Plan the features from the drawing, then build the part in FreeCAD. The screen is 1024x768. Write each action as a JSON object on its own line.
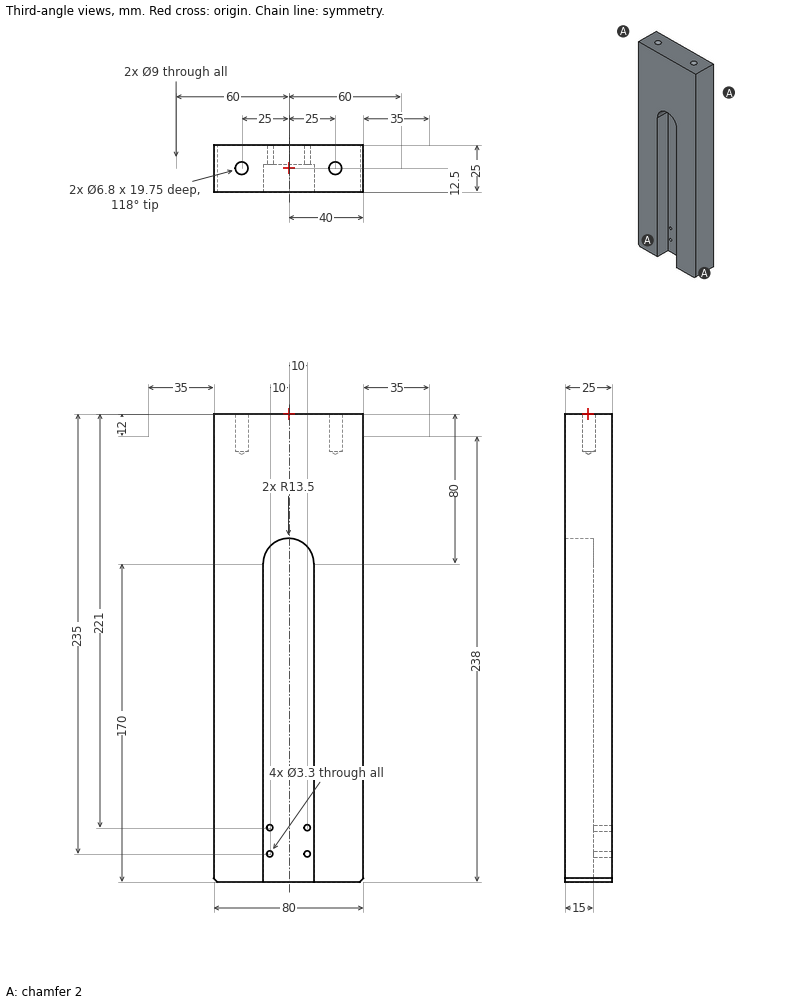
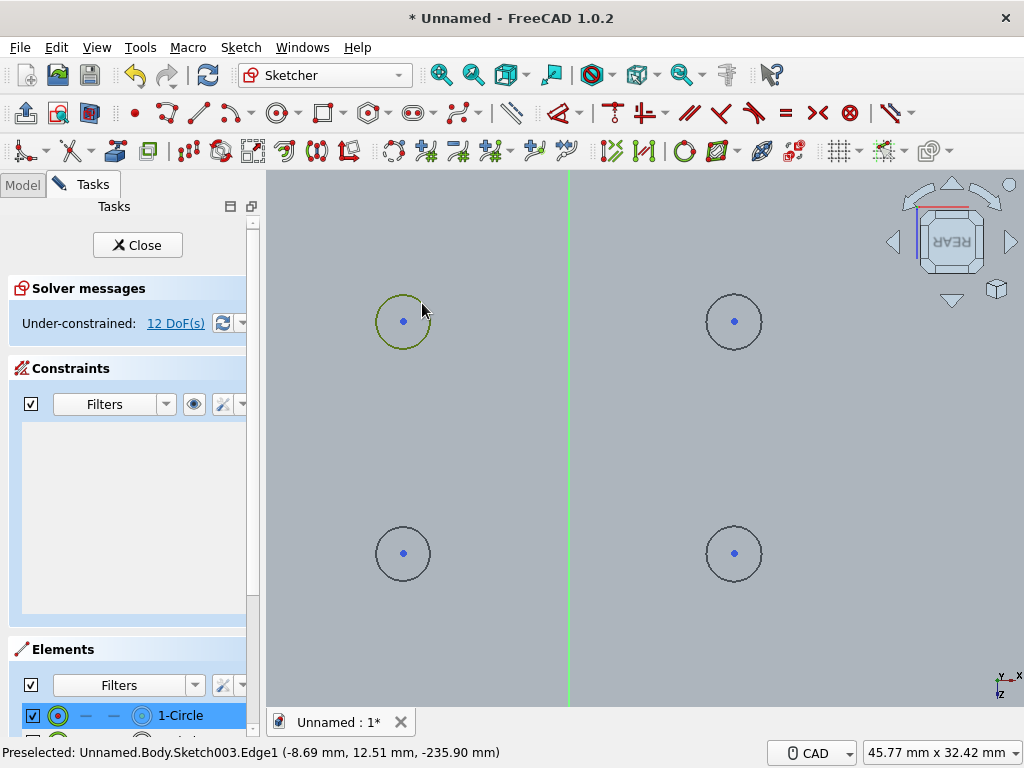
{"action": "left_click", "coordinate": [422, 535]}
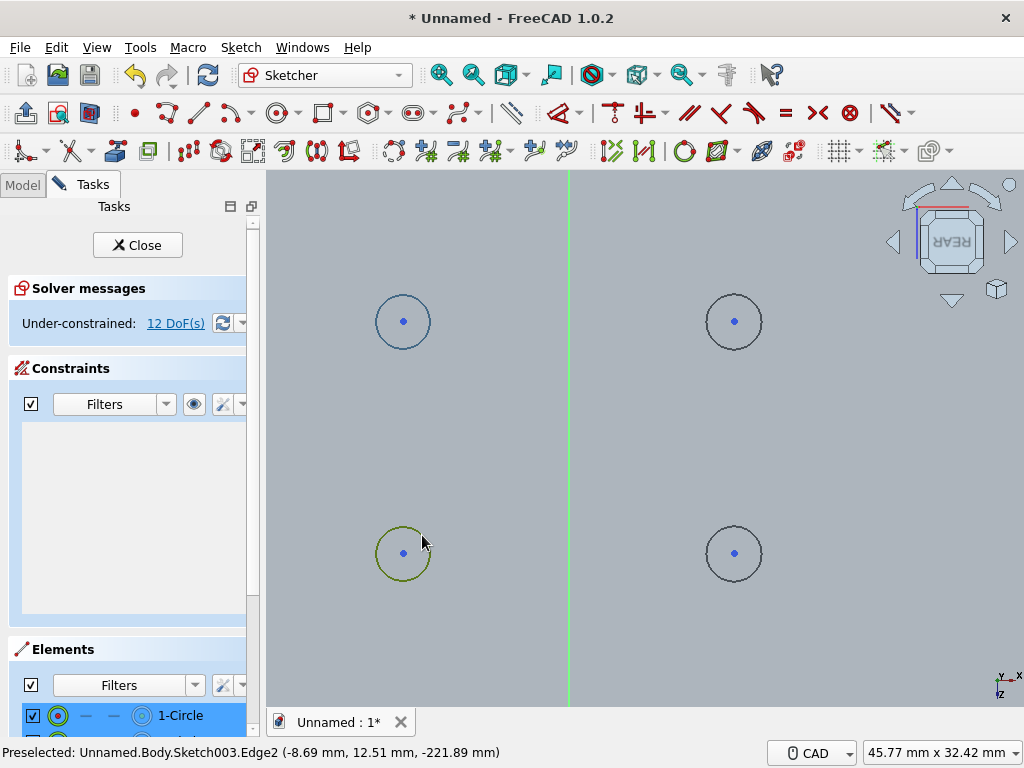
{"action": "left_click", "coordinate": [753, 534]}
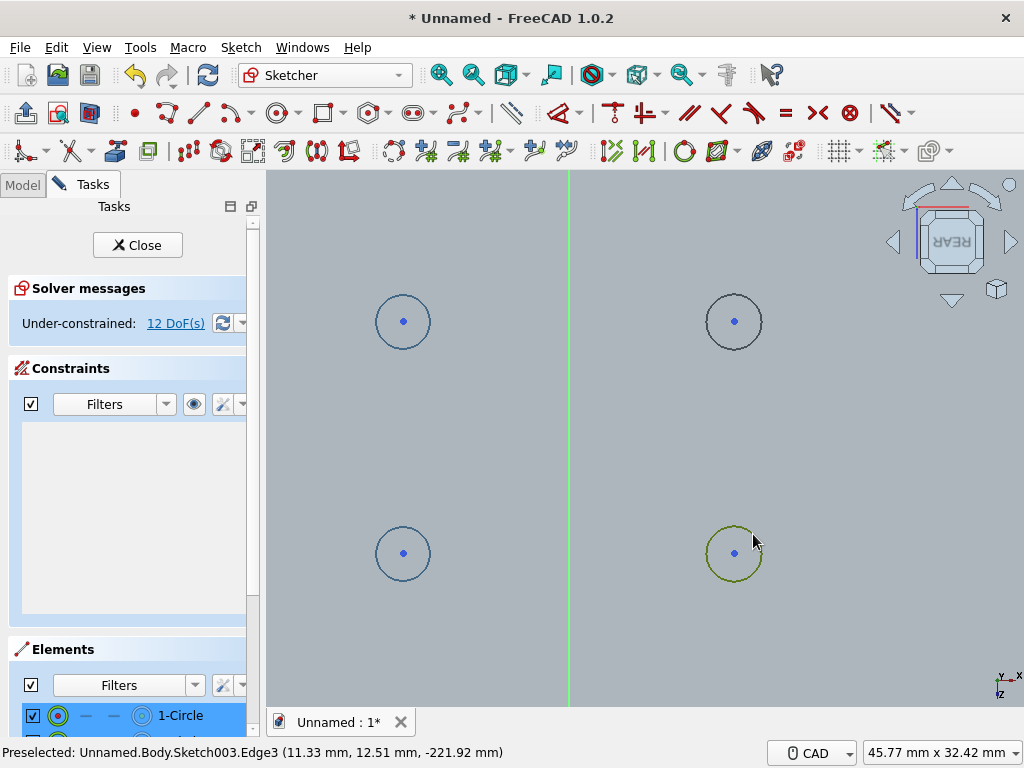
{"action": "left_click", "coordinate": [753, 302]}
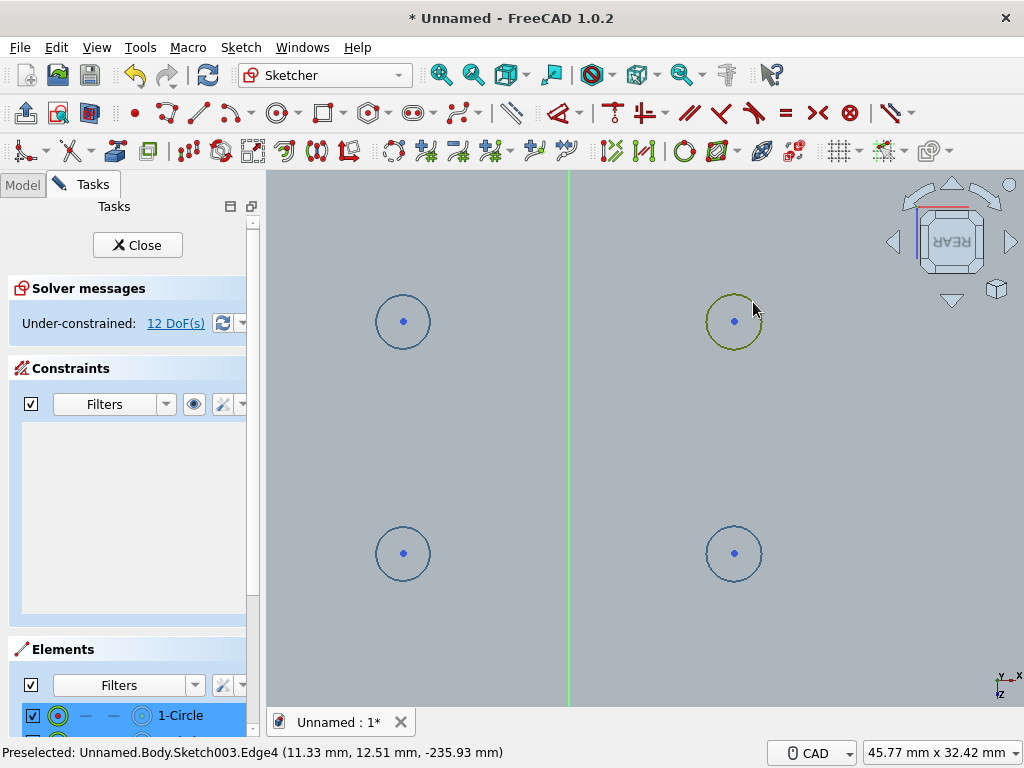
{"action": "left_click", "coordinate": [786, 114]}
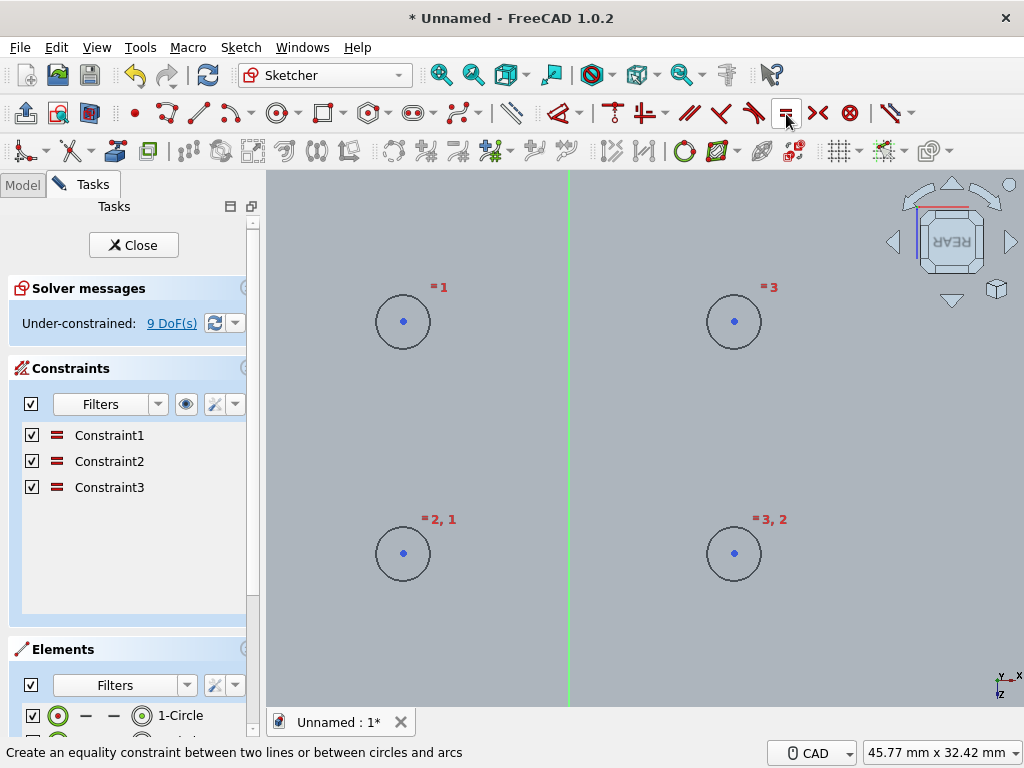
{"action": "left_click", "coordinate": [403, 322]}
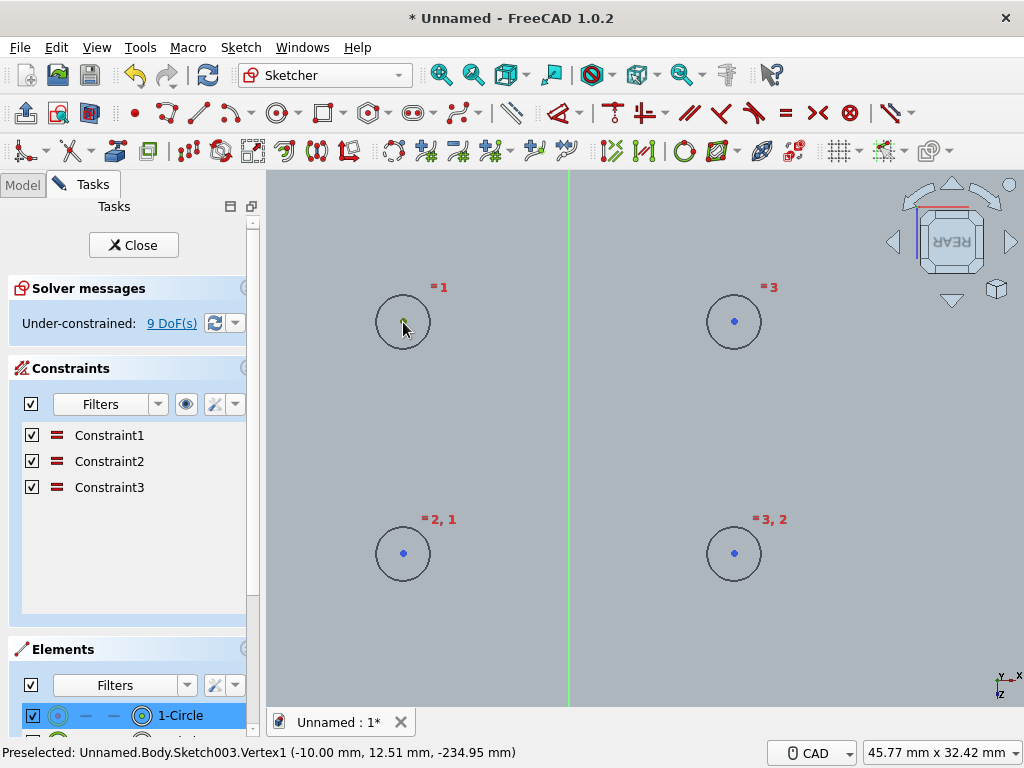
{"action": "left_click", "coordinate": [403, 554]}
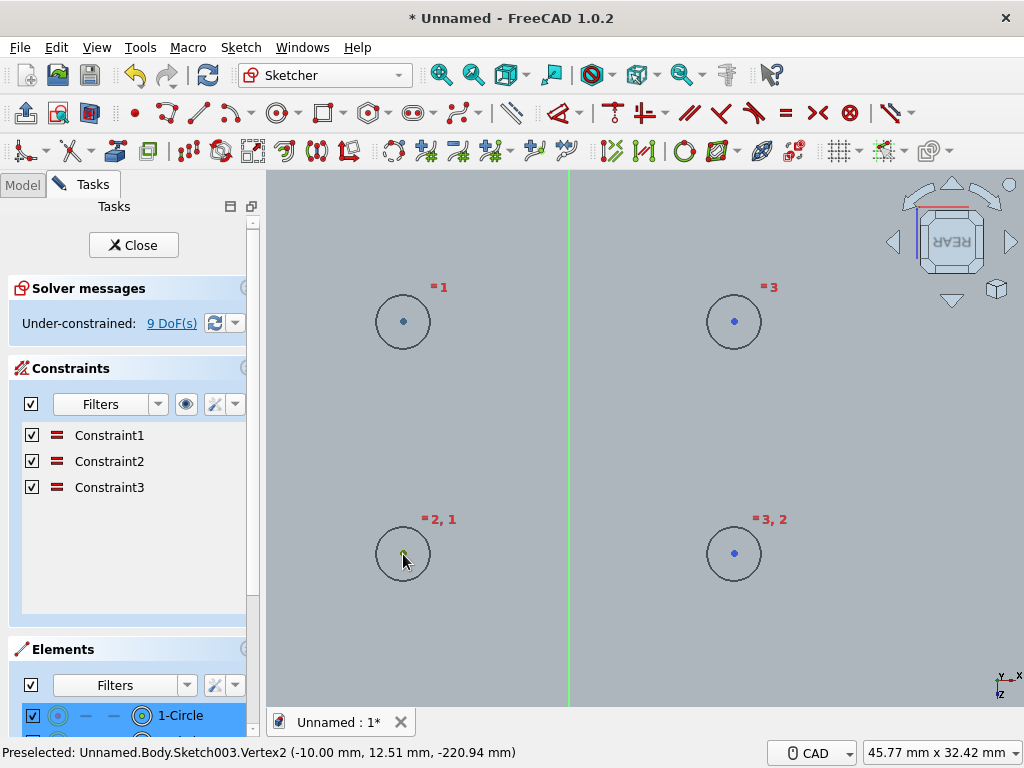
{"action": "left_click", "coordinate": [668, 114]}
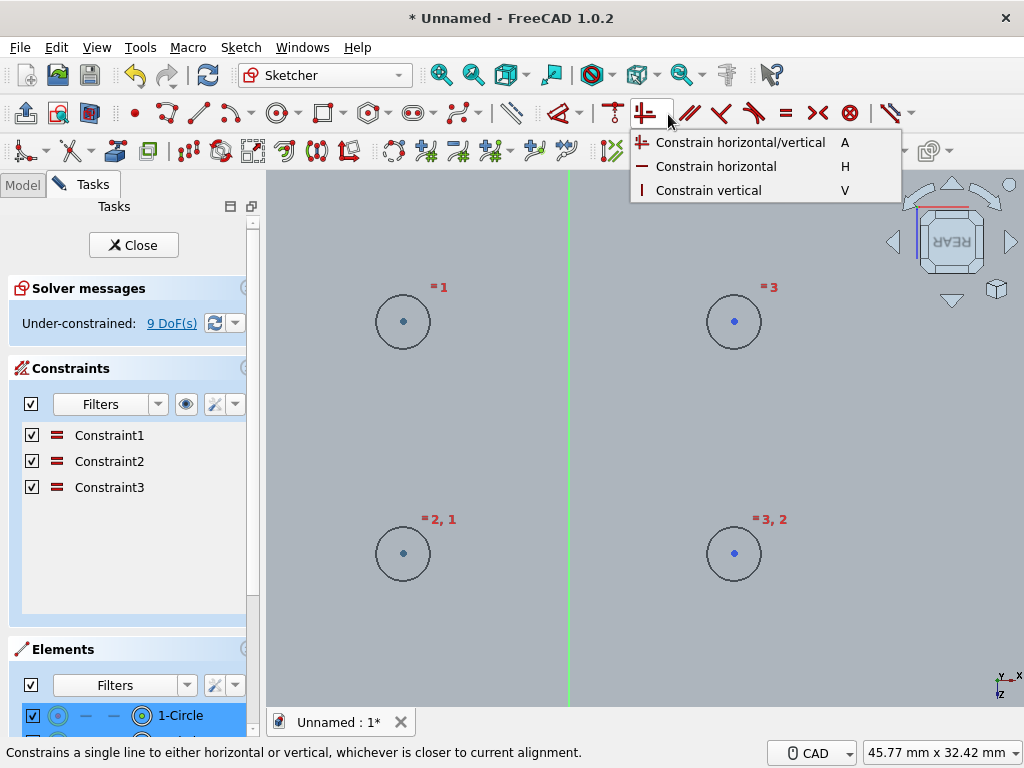
{"action": "left_click", "coordinate": [766, 190]}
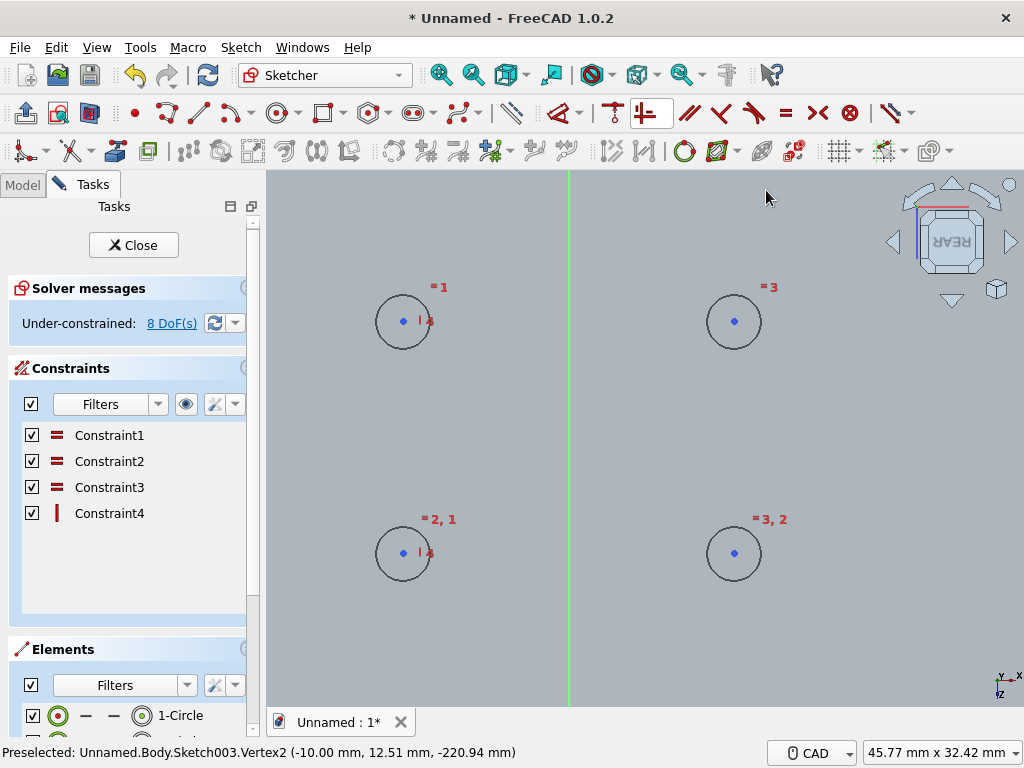
{"action": "left_click", "coordinate": [403, 554]}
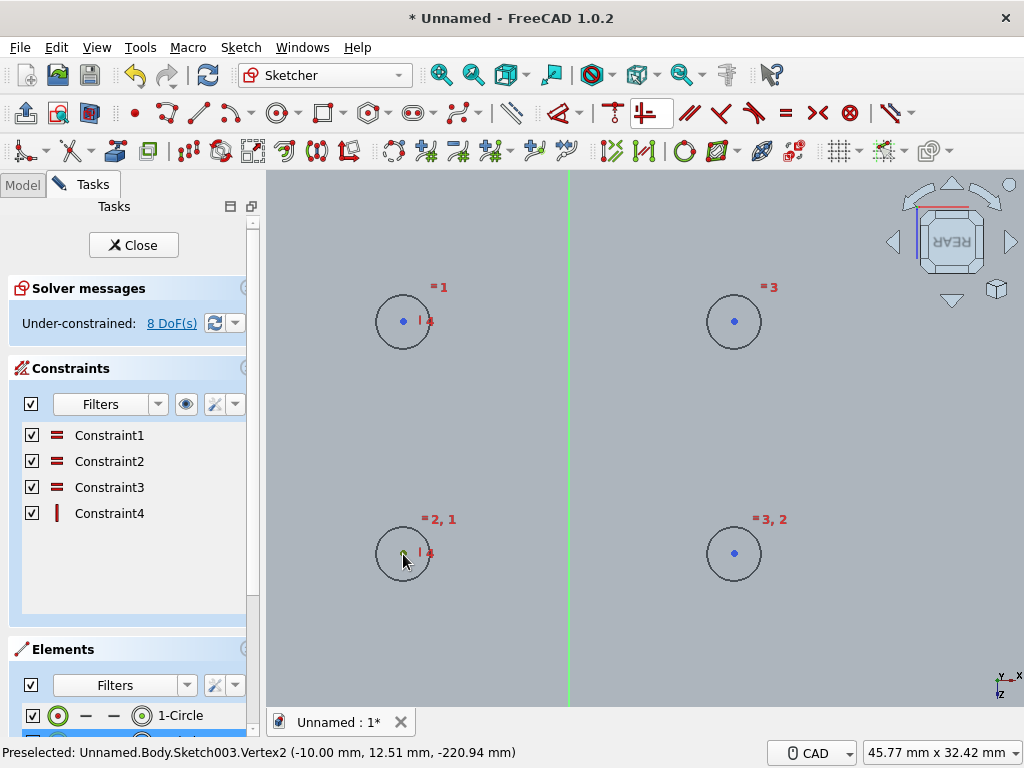
{"action": "left_click", "coordinate": [734, 554]}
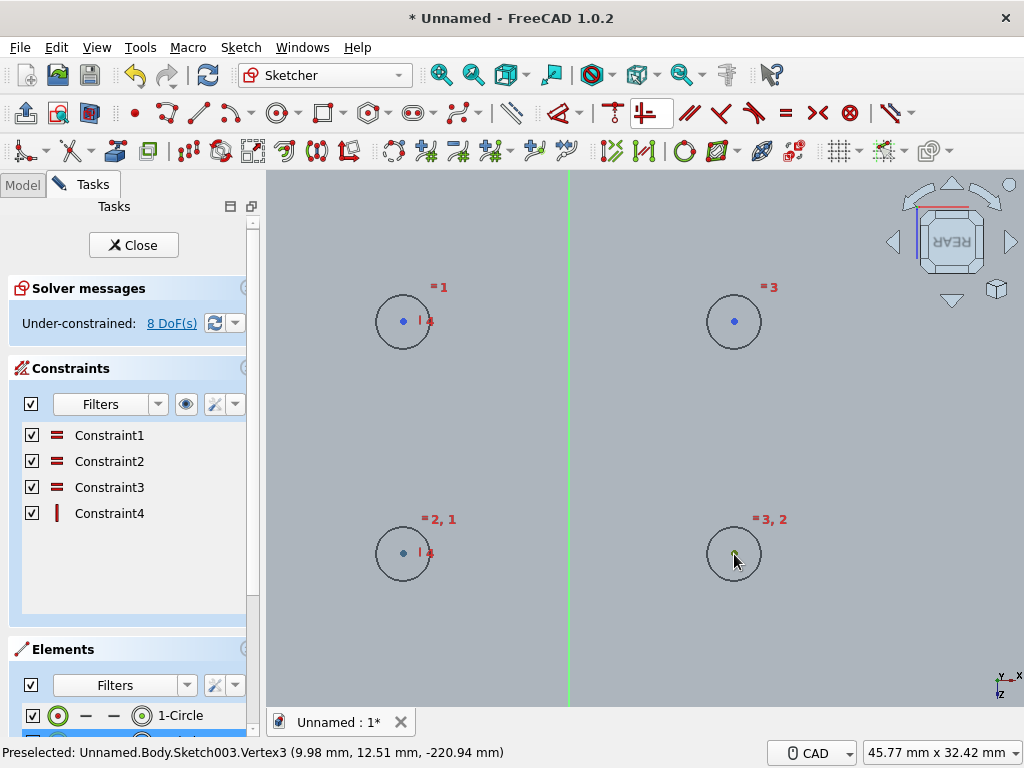
{"action": "key", "text": "h"}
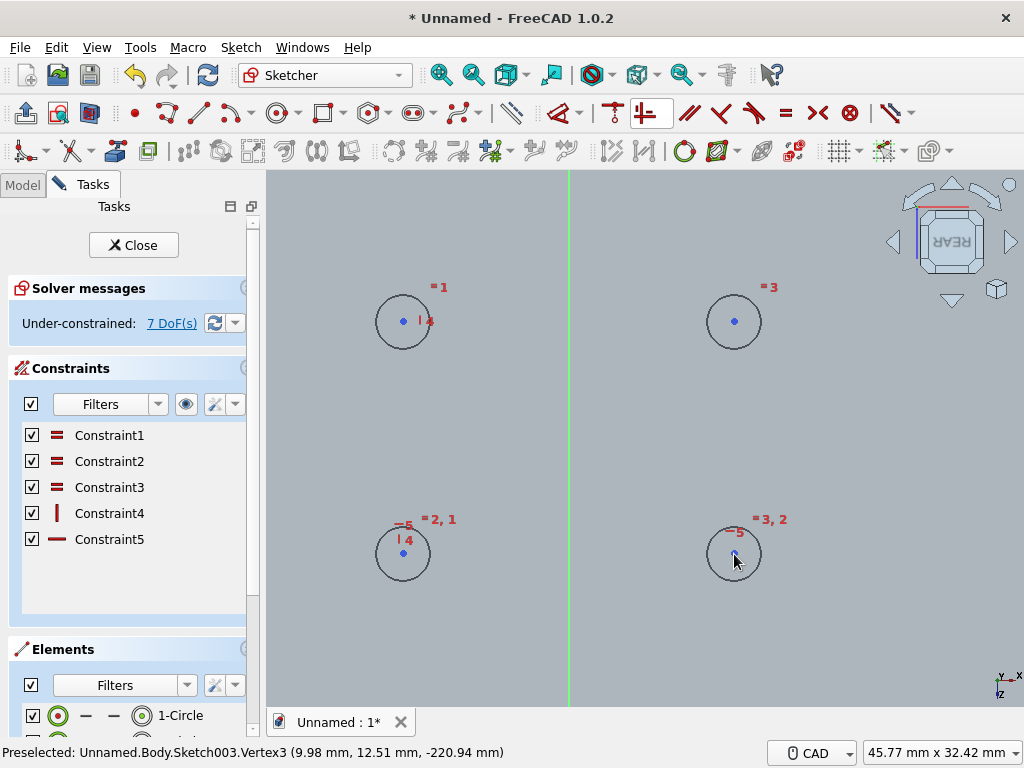
{"action": "left_click", "coordinate": [734, 554]}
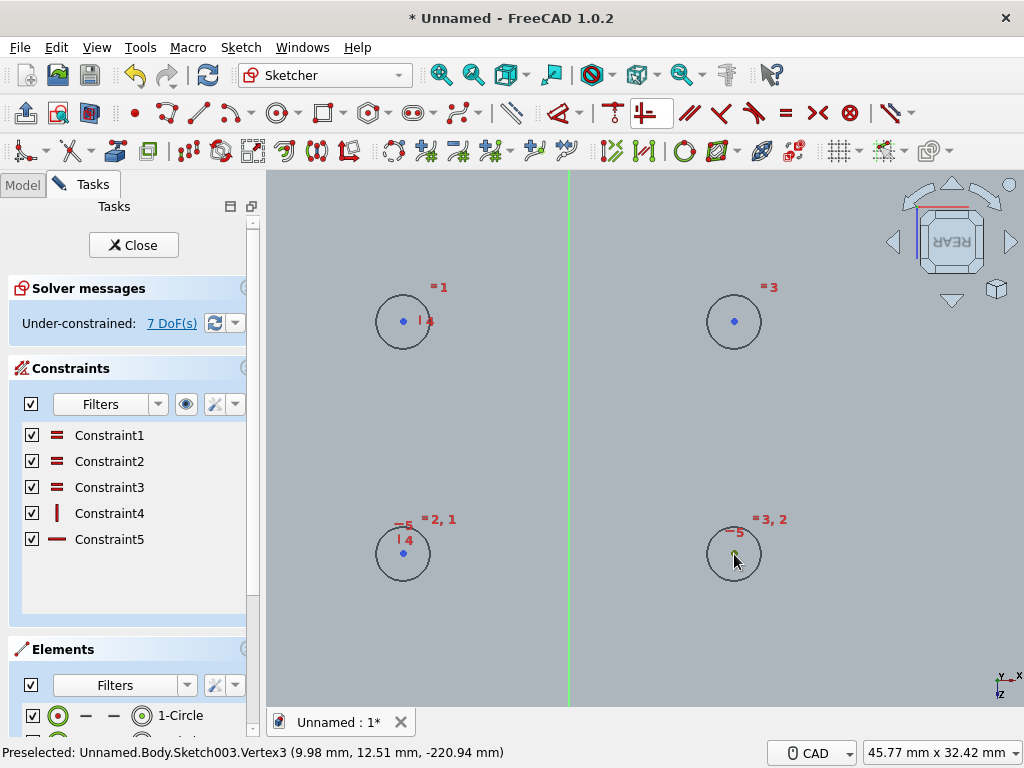
{"action": "left_click", "coordinate": [734, 322]}